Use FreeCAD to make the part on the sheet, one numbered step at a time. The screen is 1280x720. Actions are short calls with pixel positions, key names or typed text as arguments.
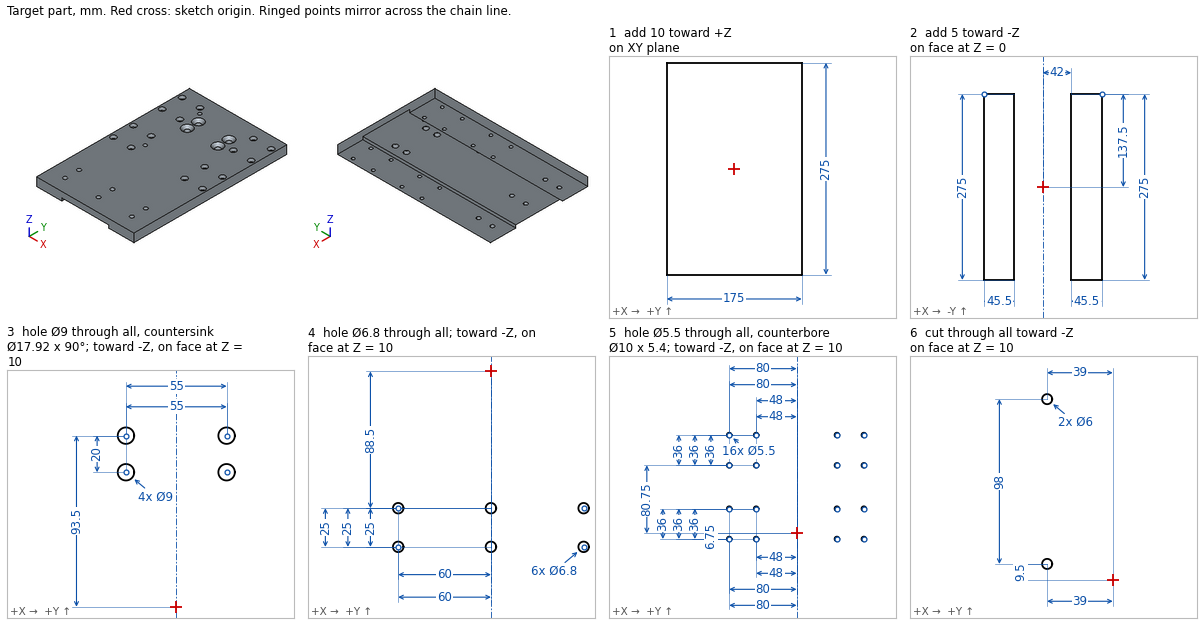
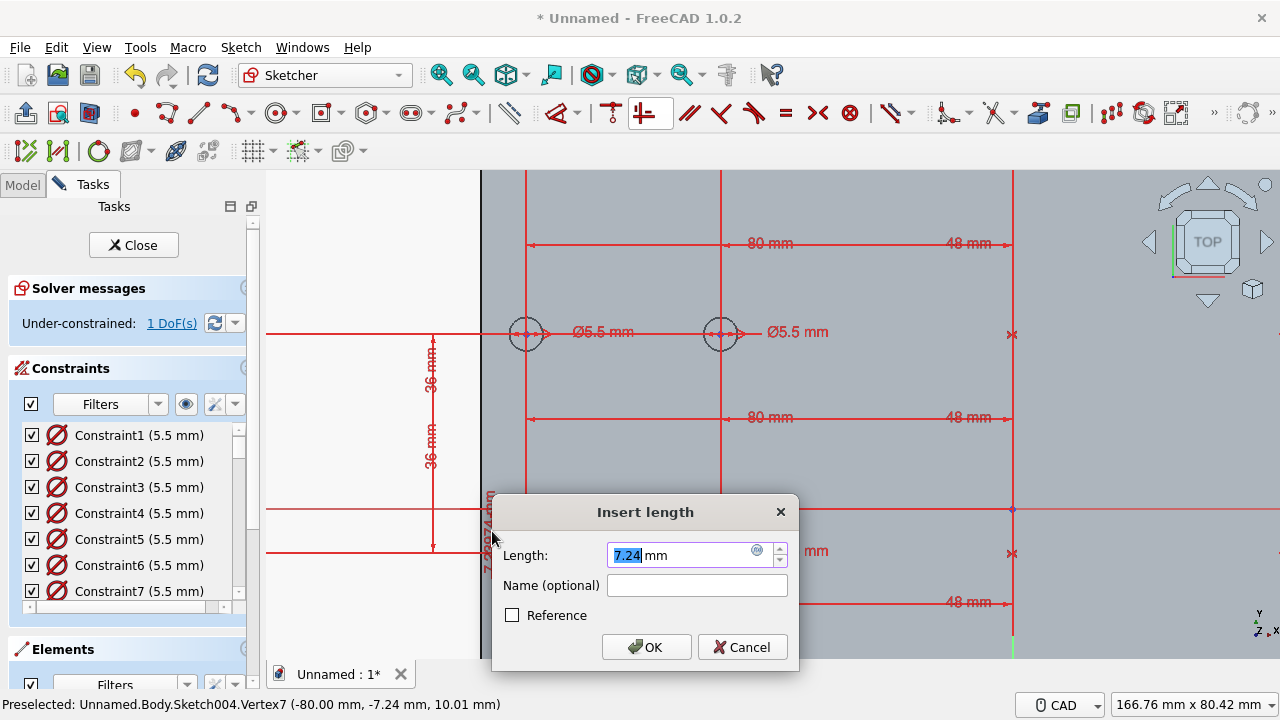
text(6.75)
key(Return)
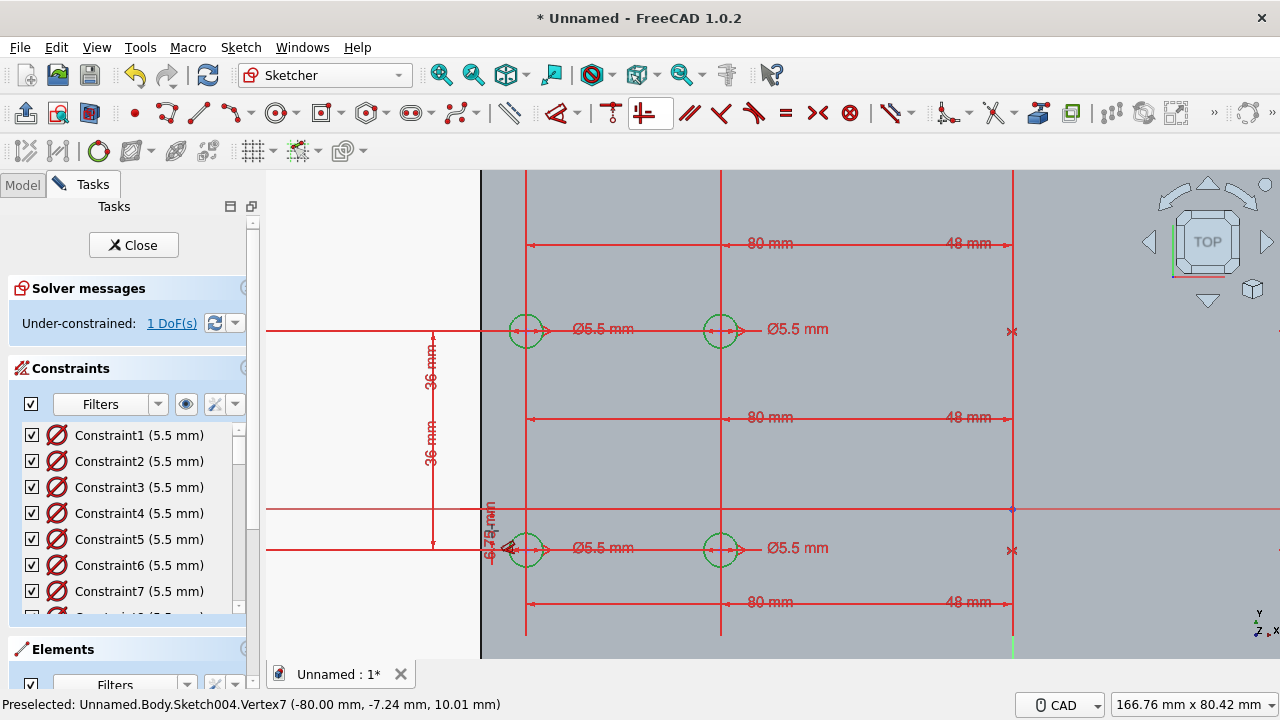
scroll(525, 554, down, 5)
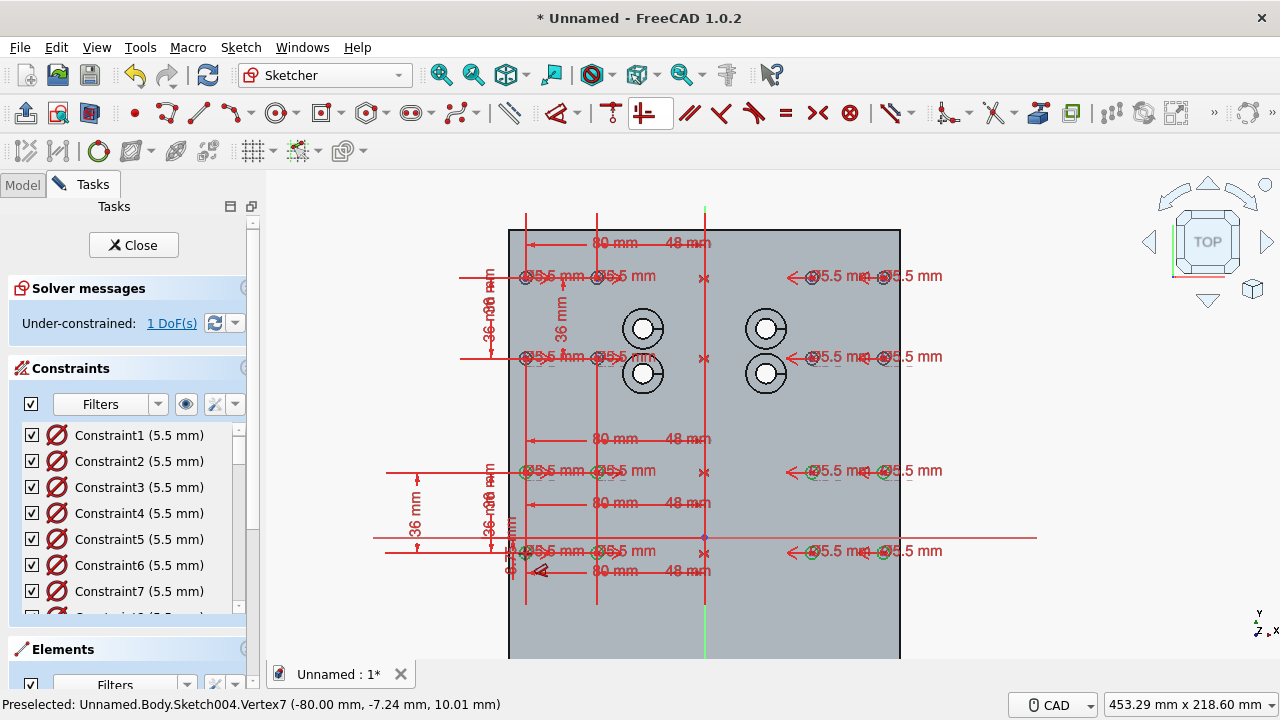
click(526, 359)
click(492, 448)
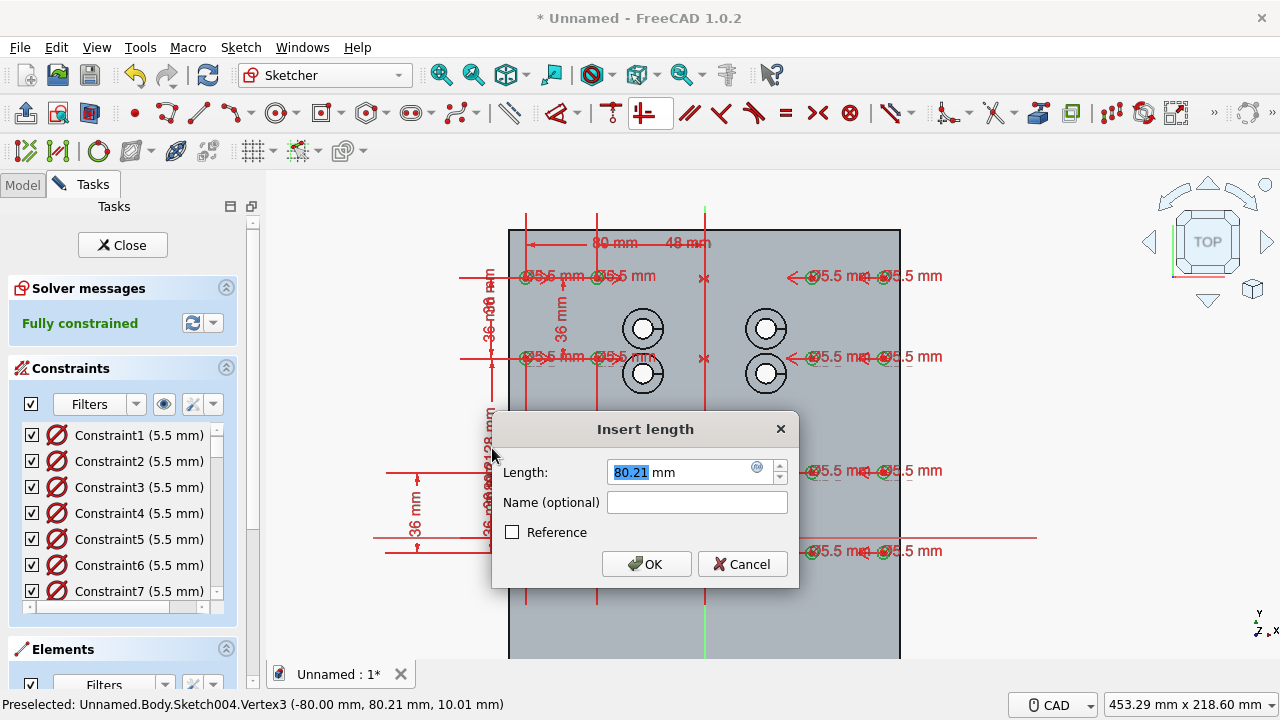
text(80.75)
key(Return)
key(Escape)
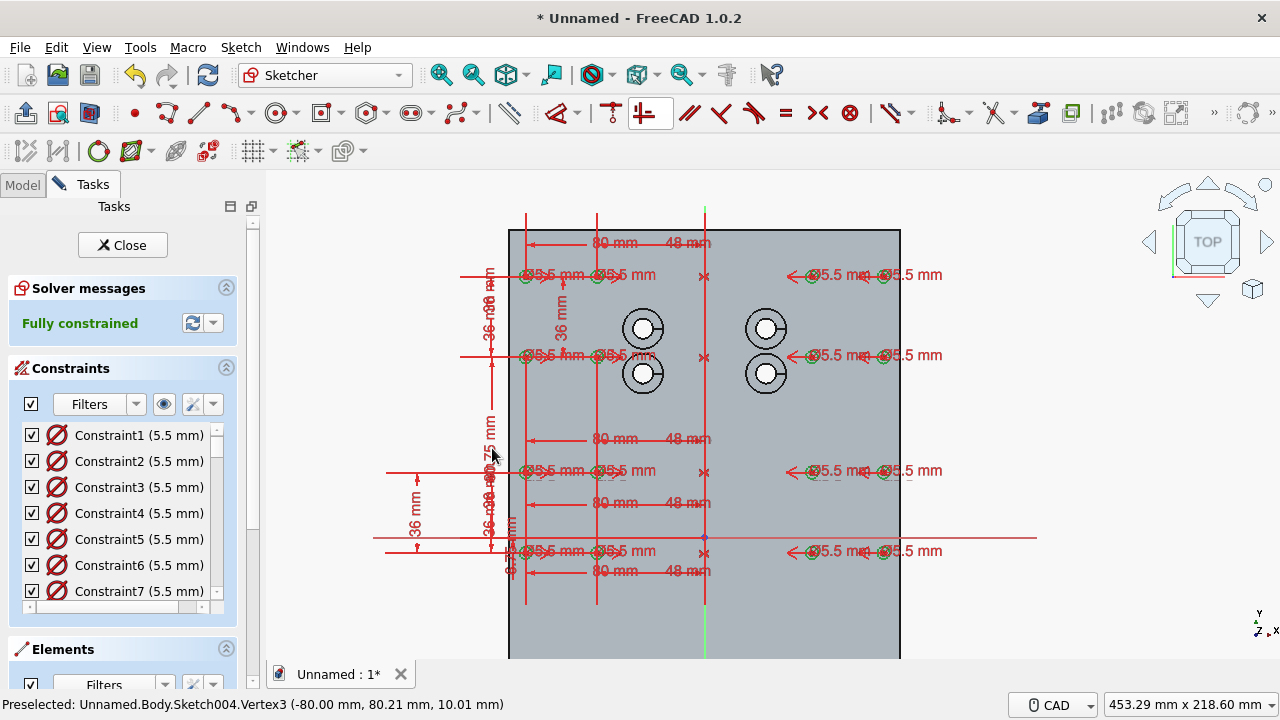
click(123, 245)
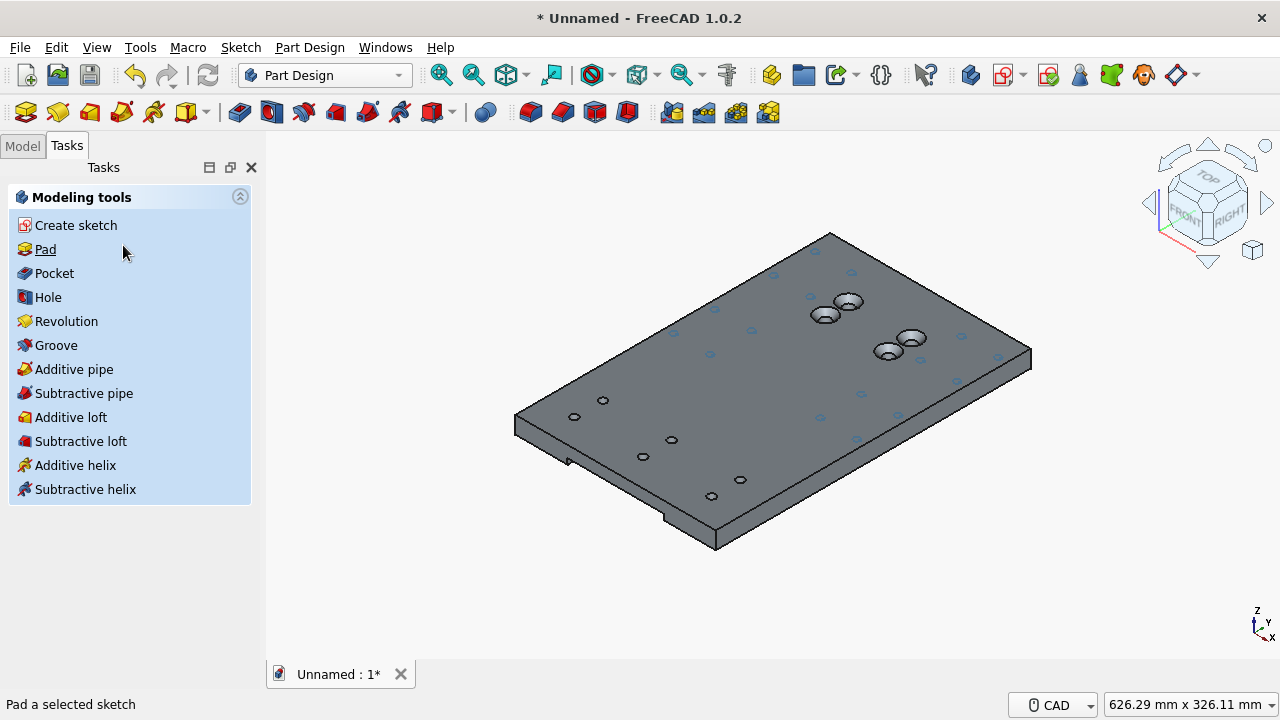
click(272, 112)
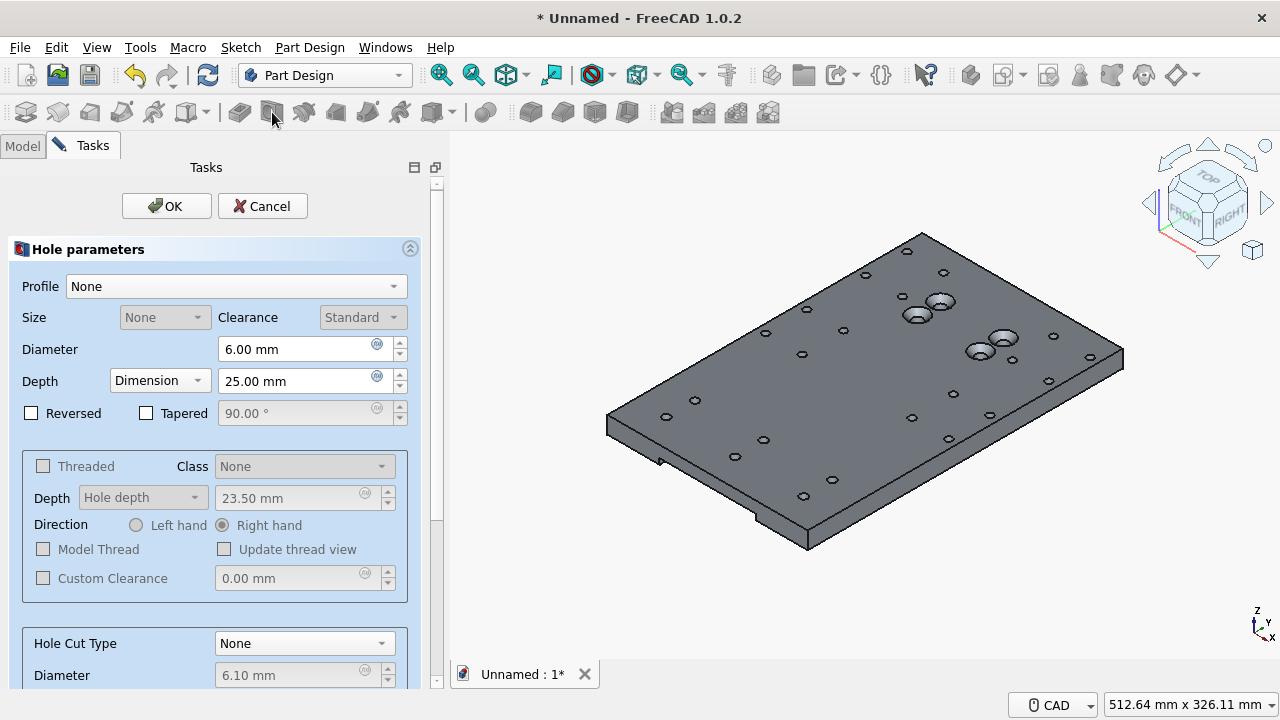
triple_click(305, 349)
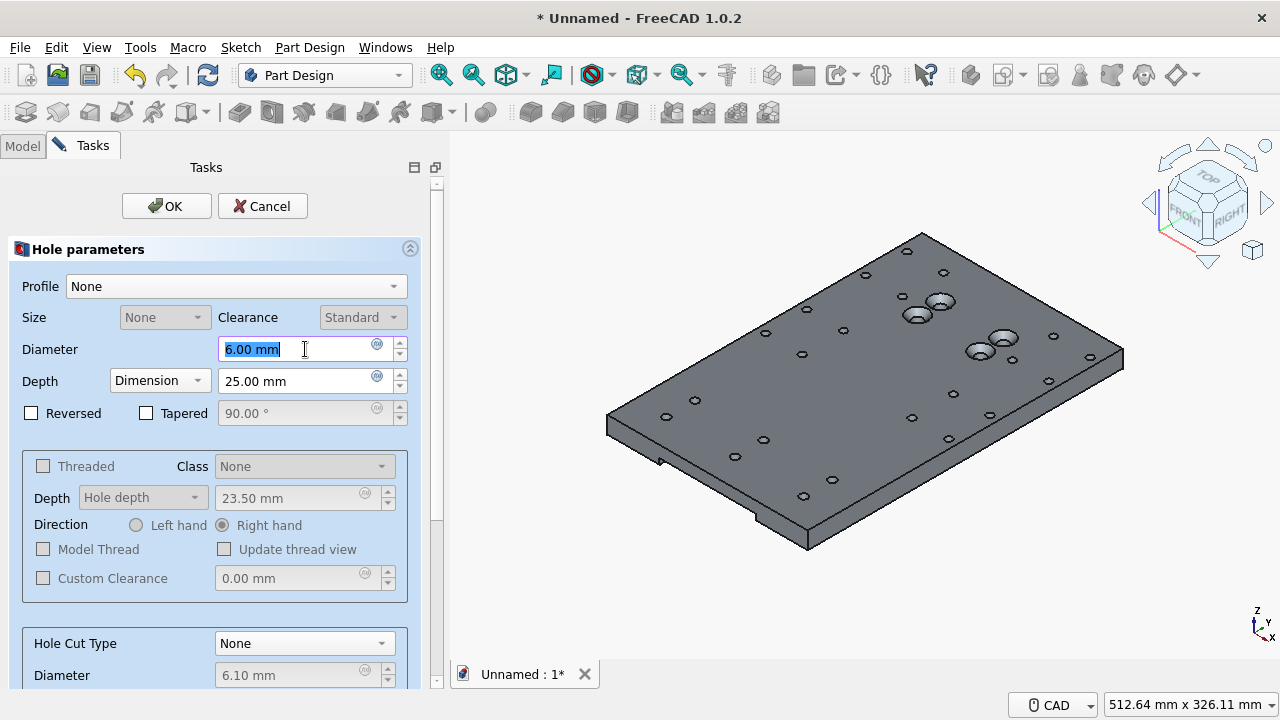
text(5.5)
key(Tab)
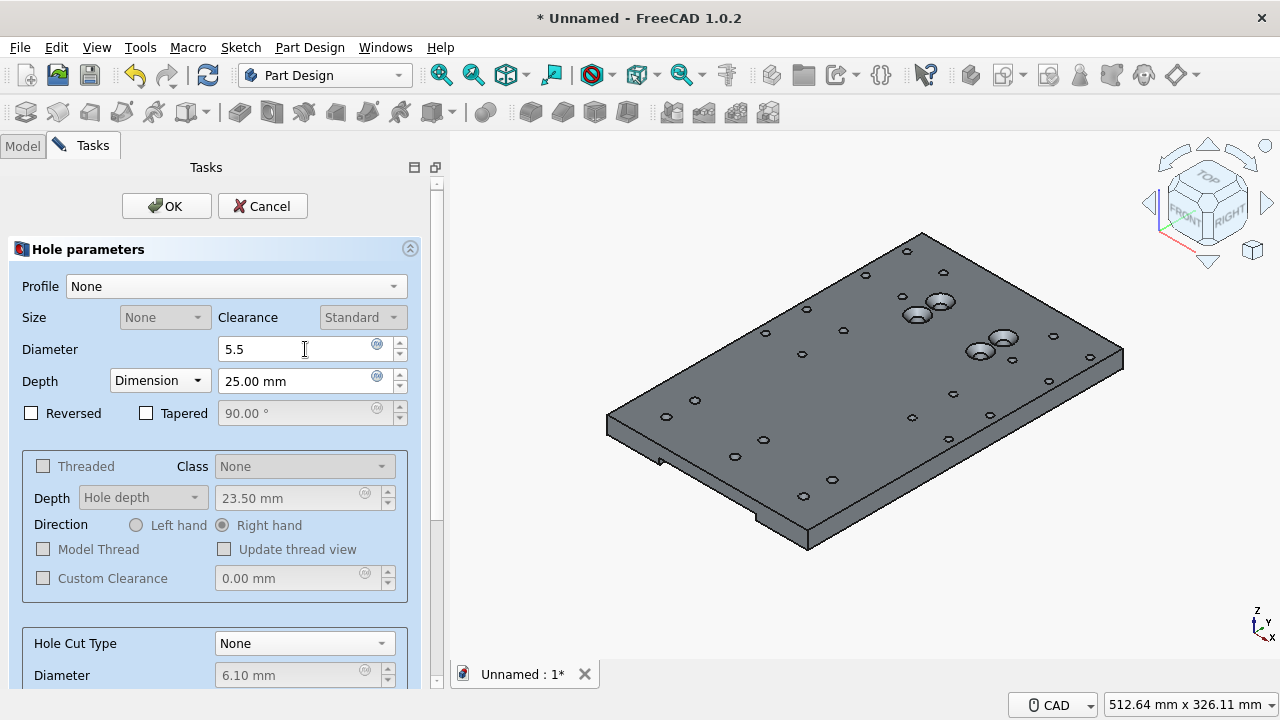
click(161, 380)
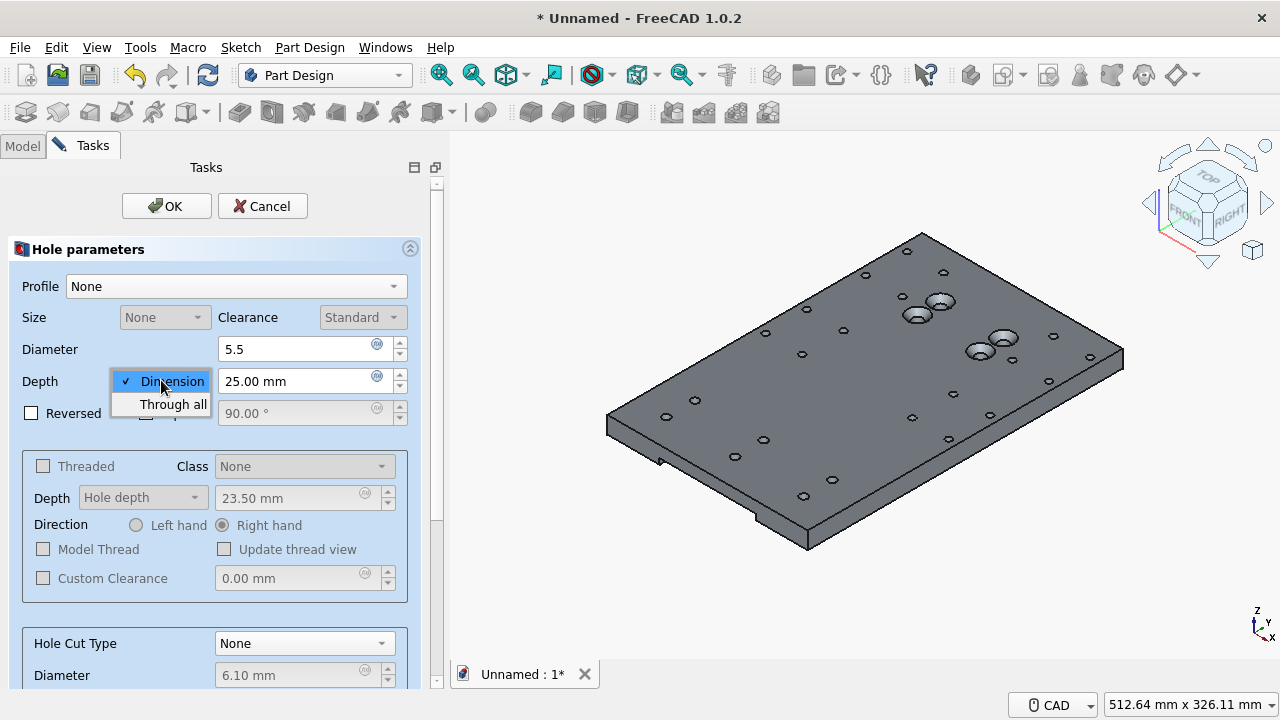
click(160, 404)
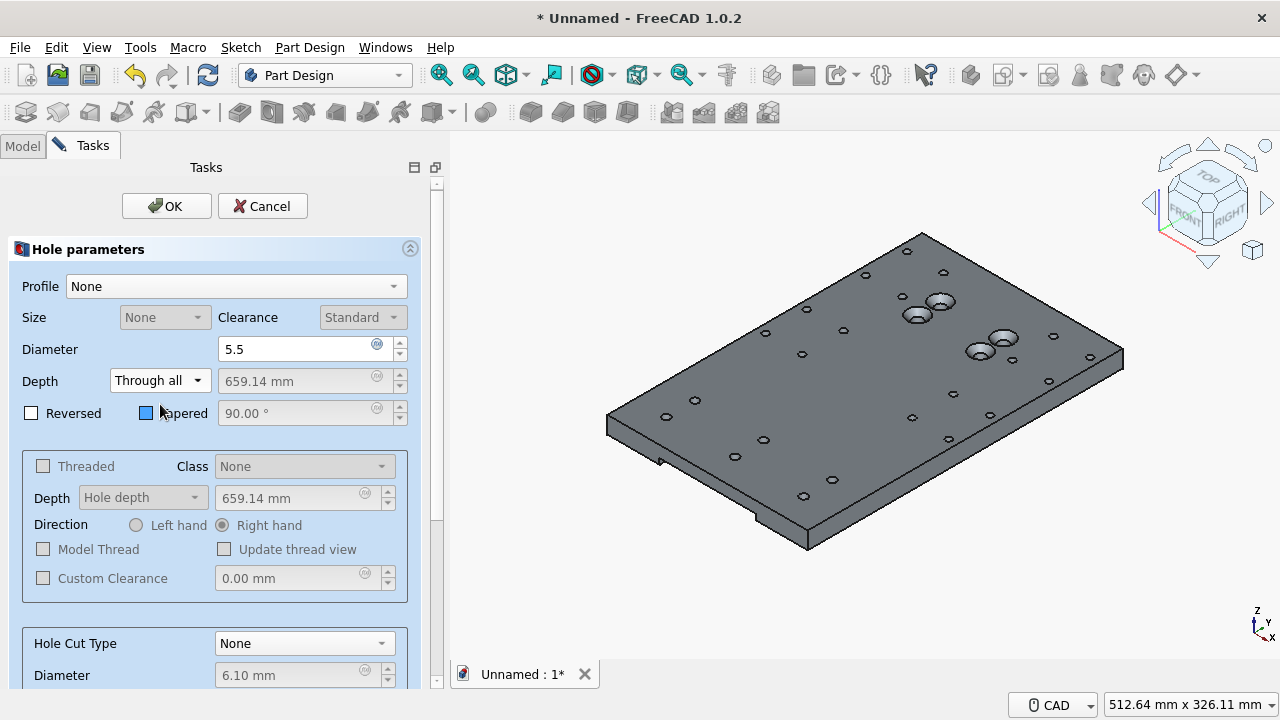
click(306, 644)